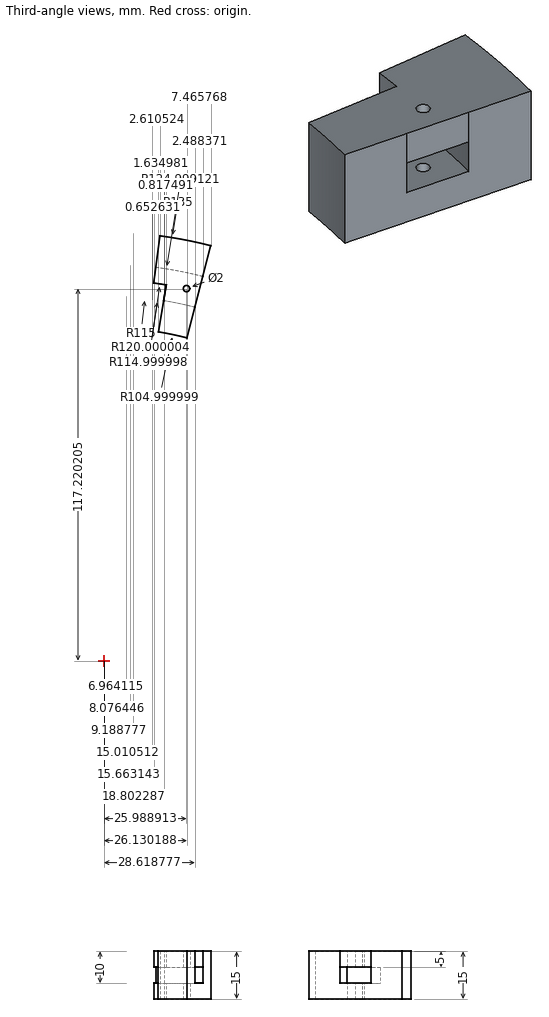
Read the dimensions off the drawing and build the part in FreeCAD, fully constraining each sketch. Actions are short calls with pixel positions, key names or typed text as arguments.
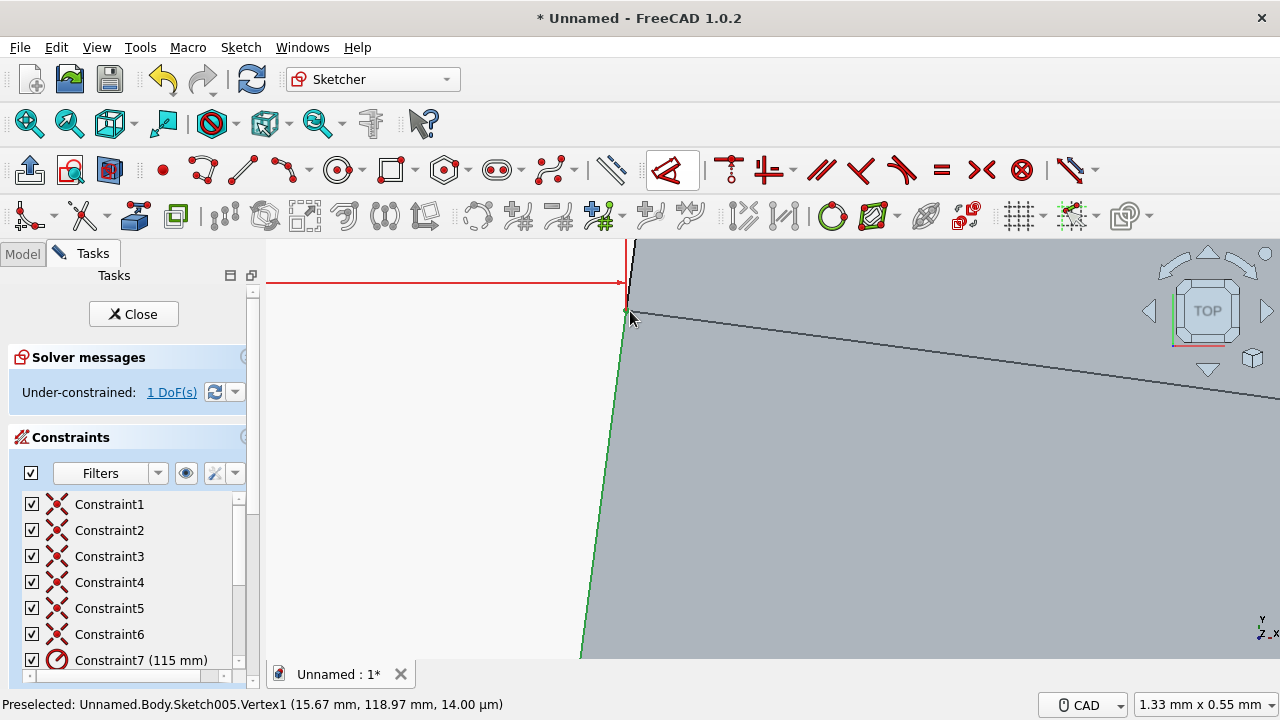
scroll(628, 322, down, 14)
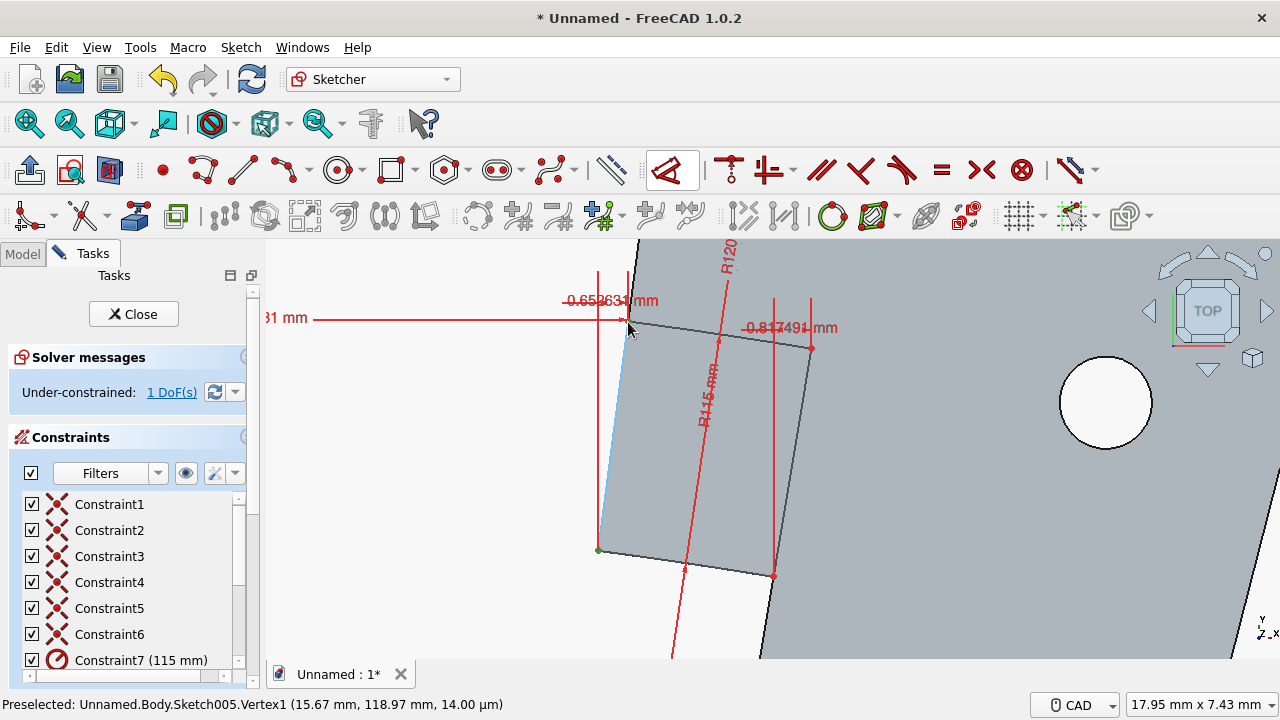
scroll(774, 577, up, 14)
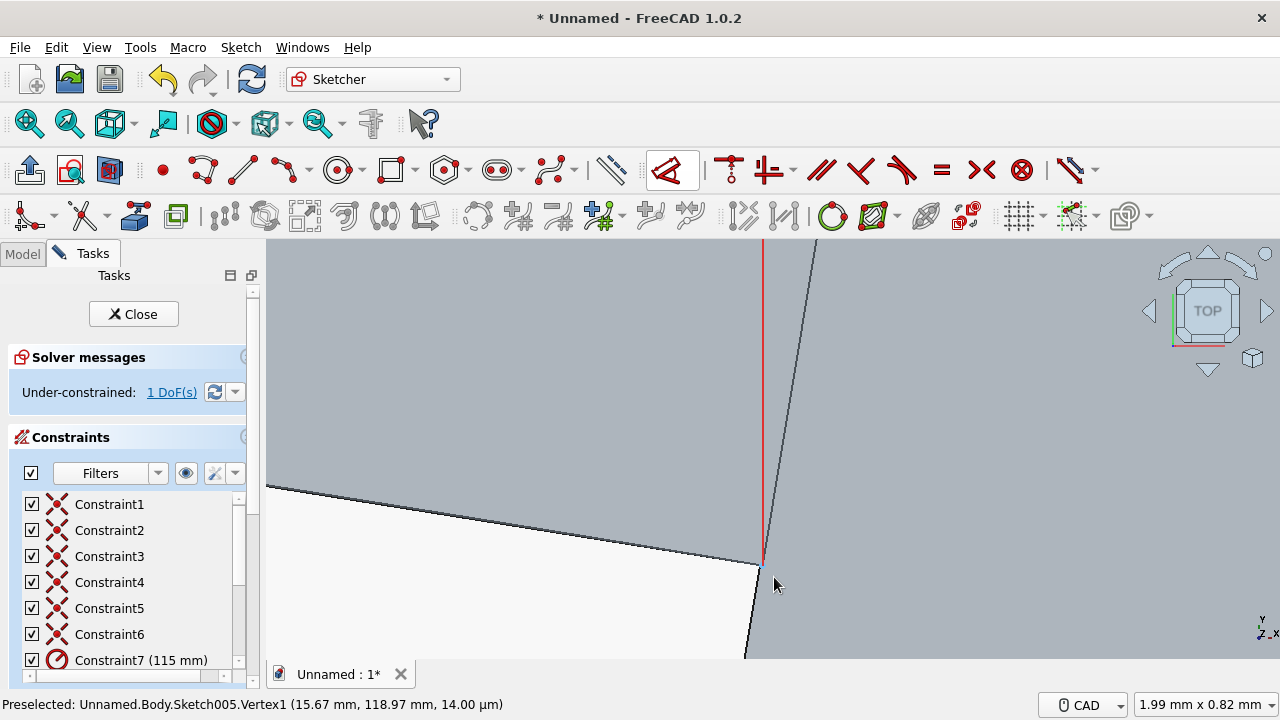
click(760, 563)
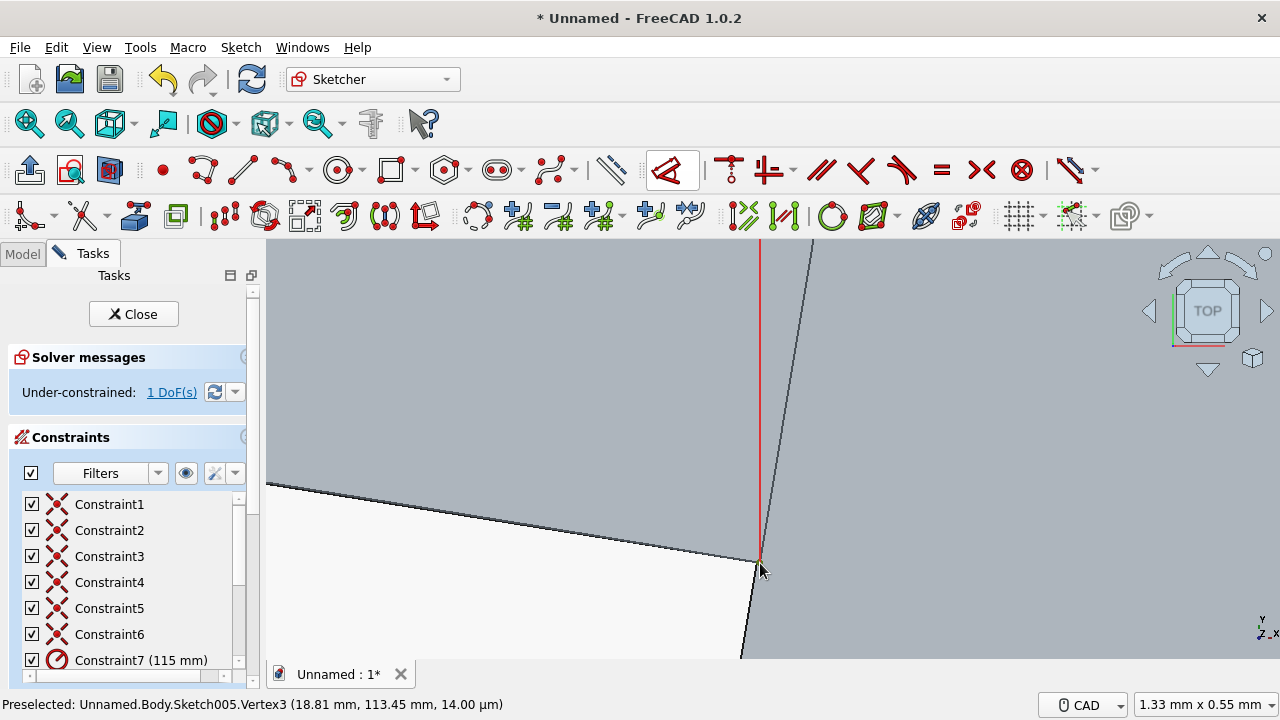
click(694, 170)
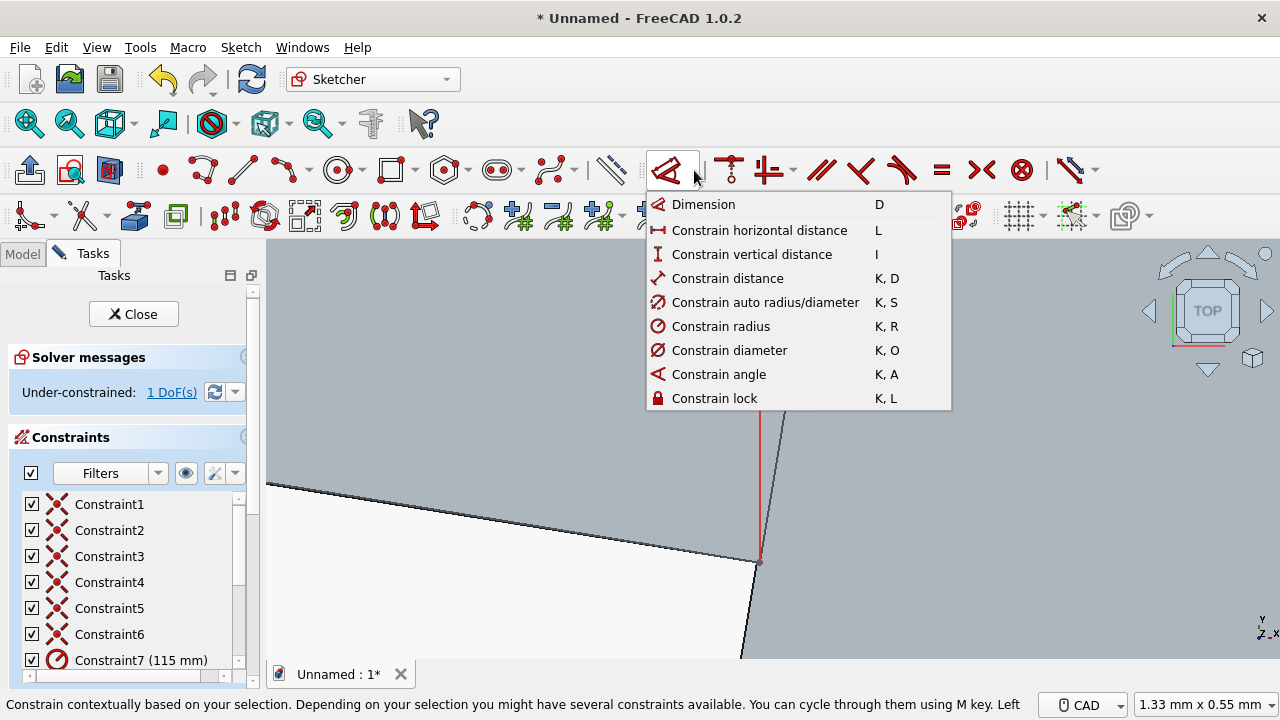
click(799, 230)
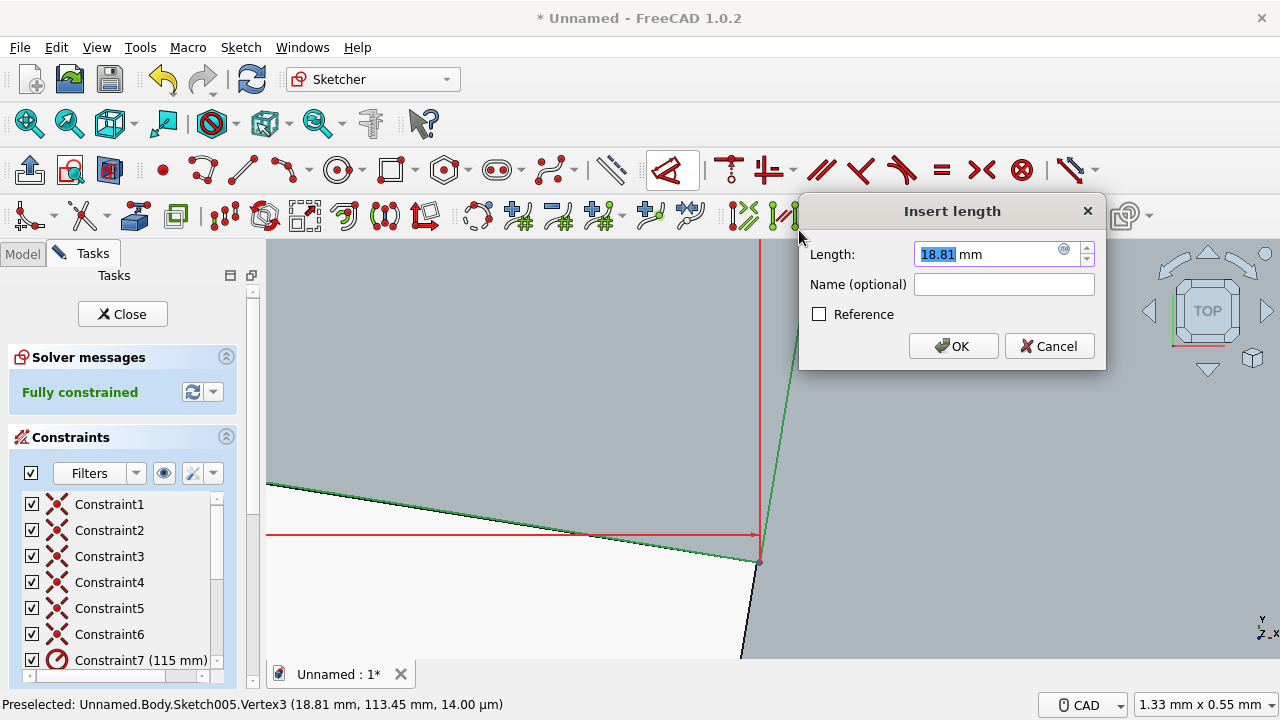
text(18.802287)
key(Return)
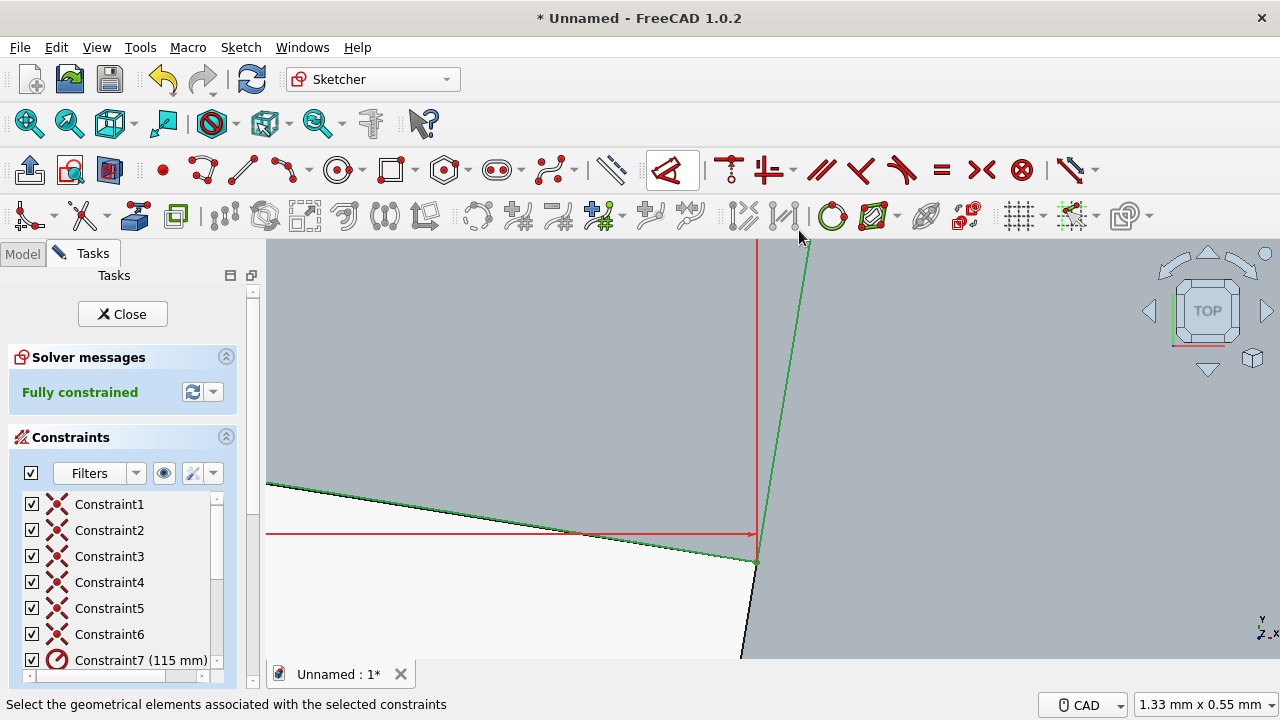
click(123, 314)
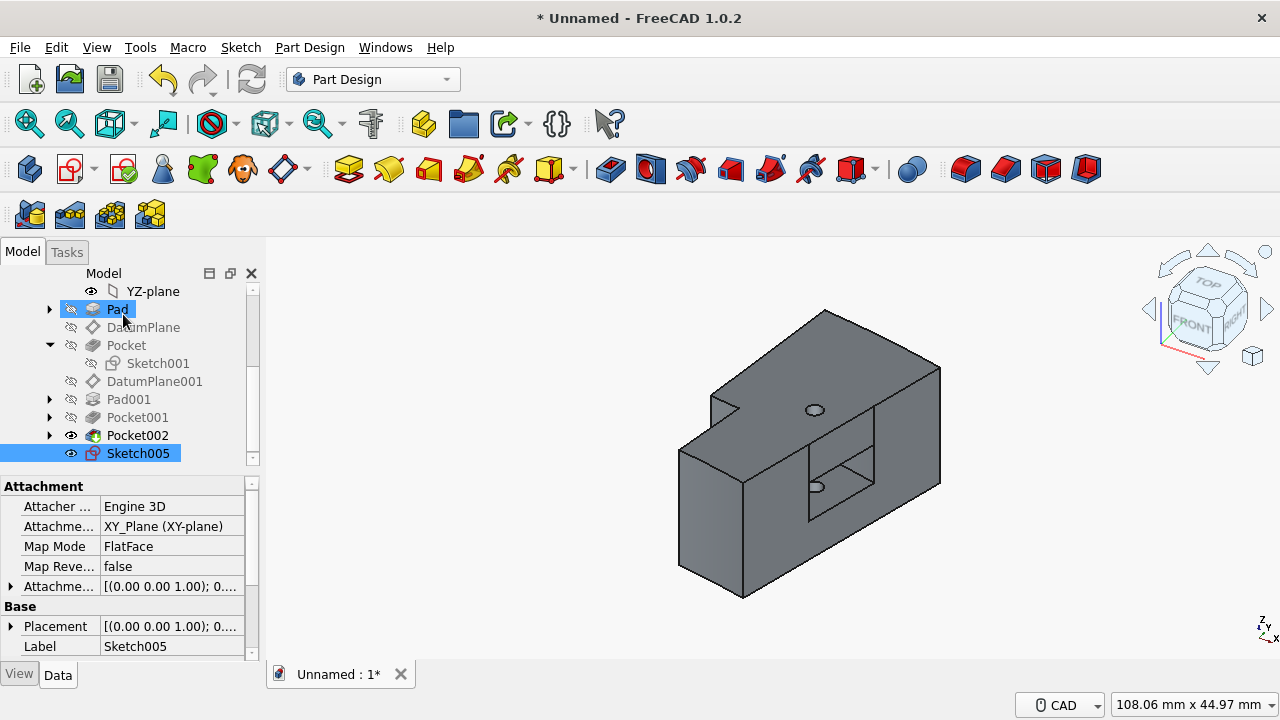
click(612, 170)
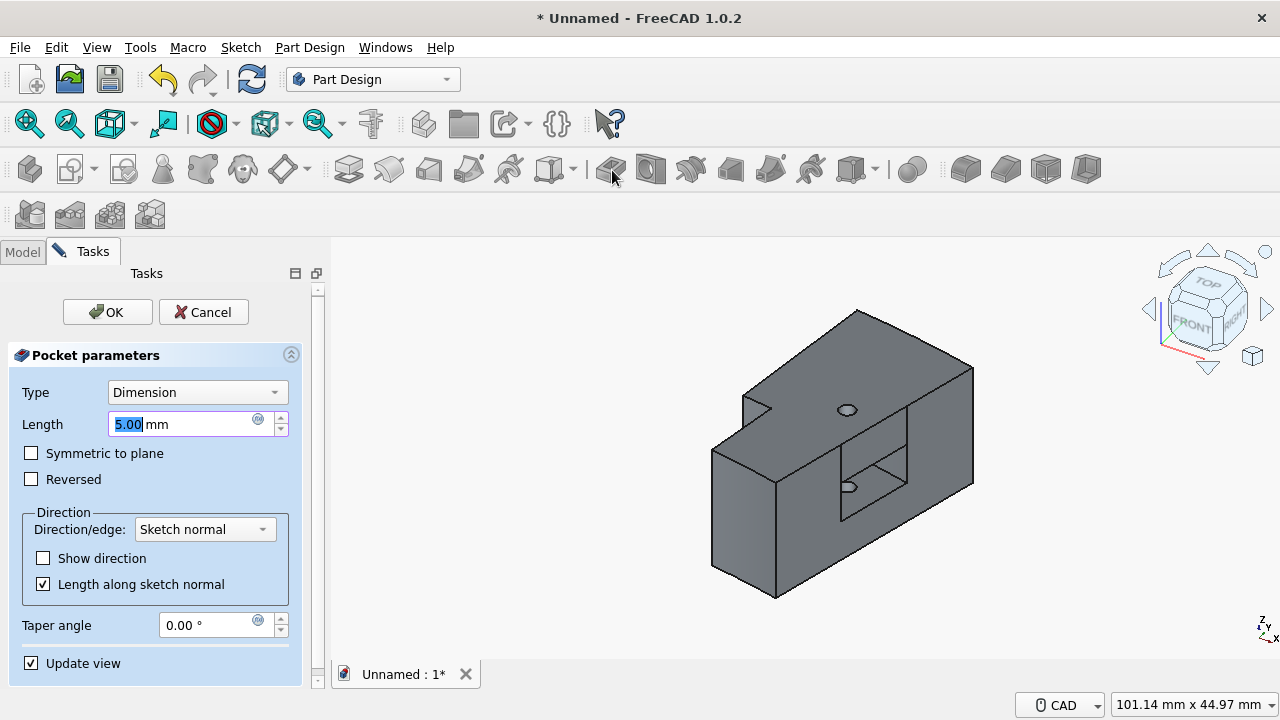
text(15)
key(Tab)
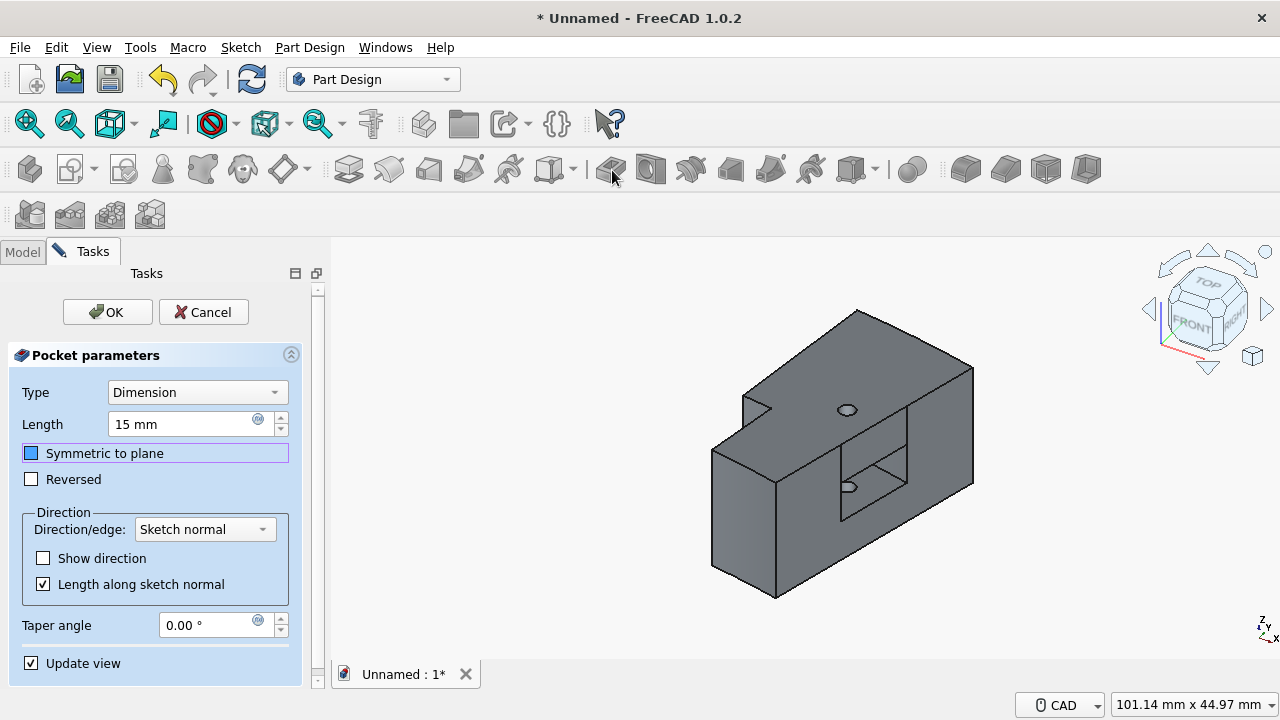
click(30, 479)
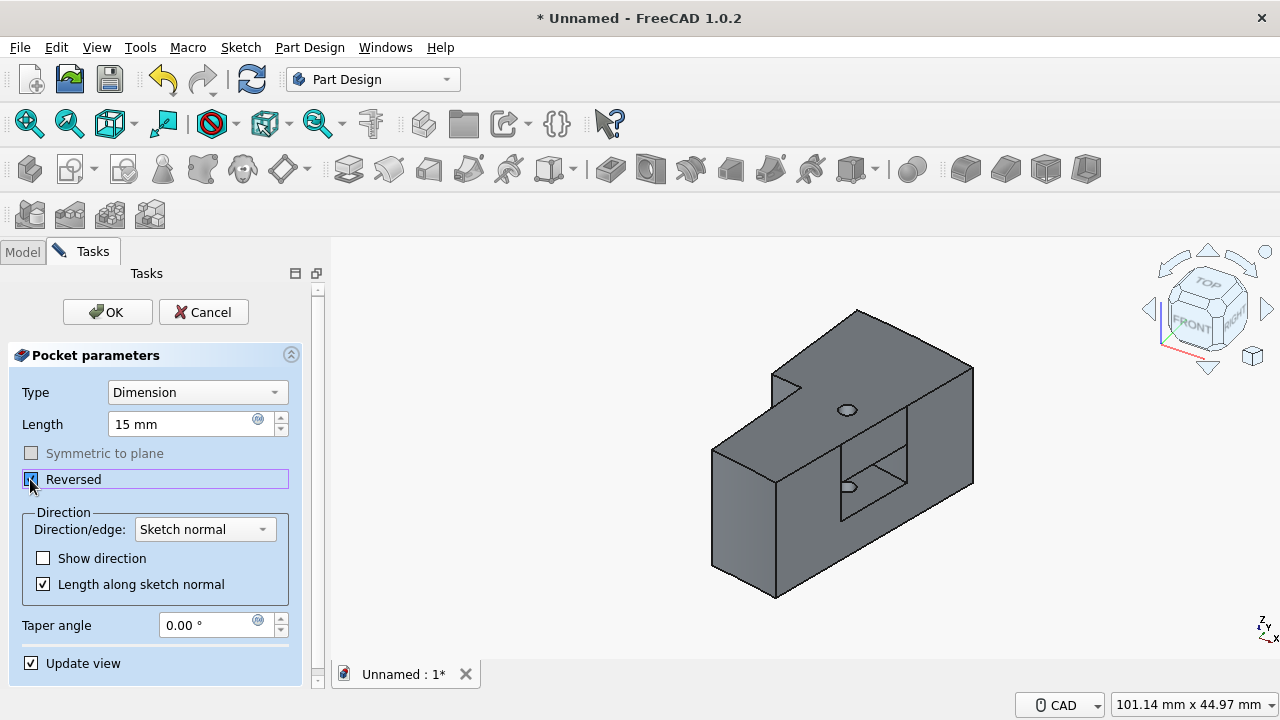
click(108, 312)